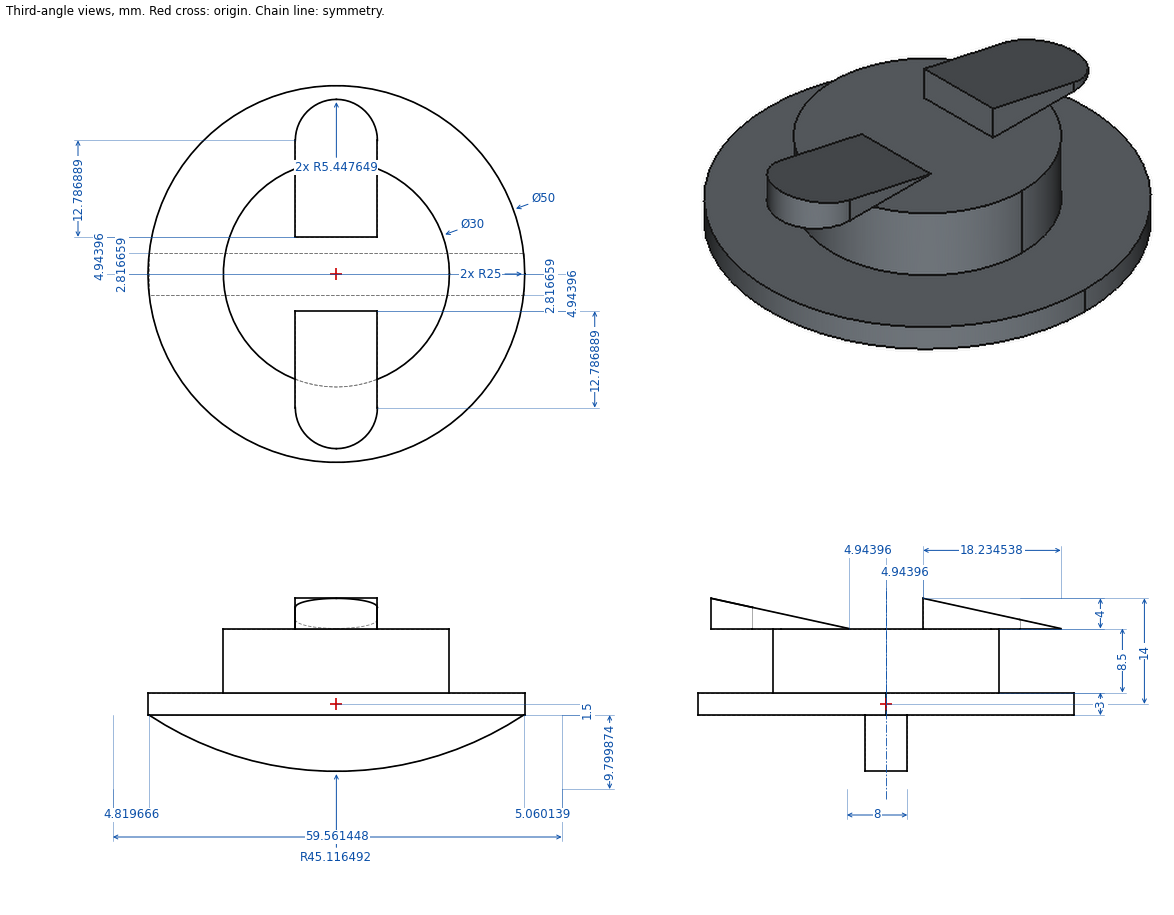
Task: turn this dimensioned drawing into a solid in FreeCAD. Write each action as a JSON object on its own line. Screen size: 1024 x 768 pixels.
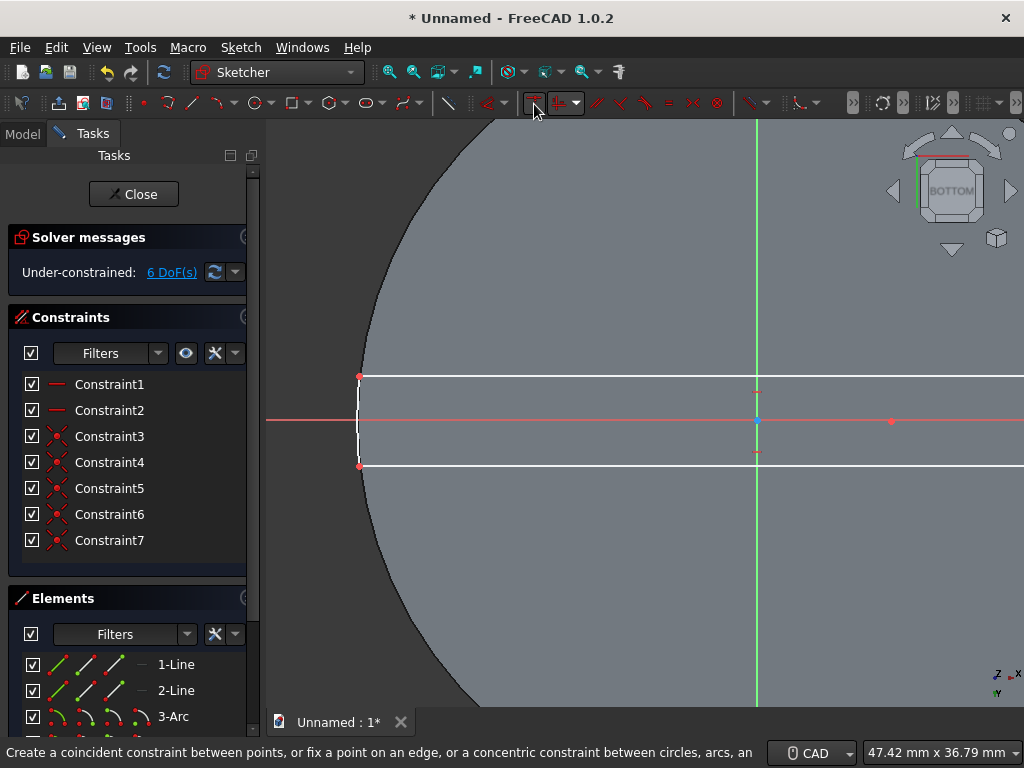
{"action": "left_click_drag", "start_coordinate": [747, 410], "coordinate": [901, 431]}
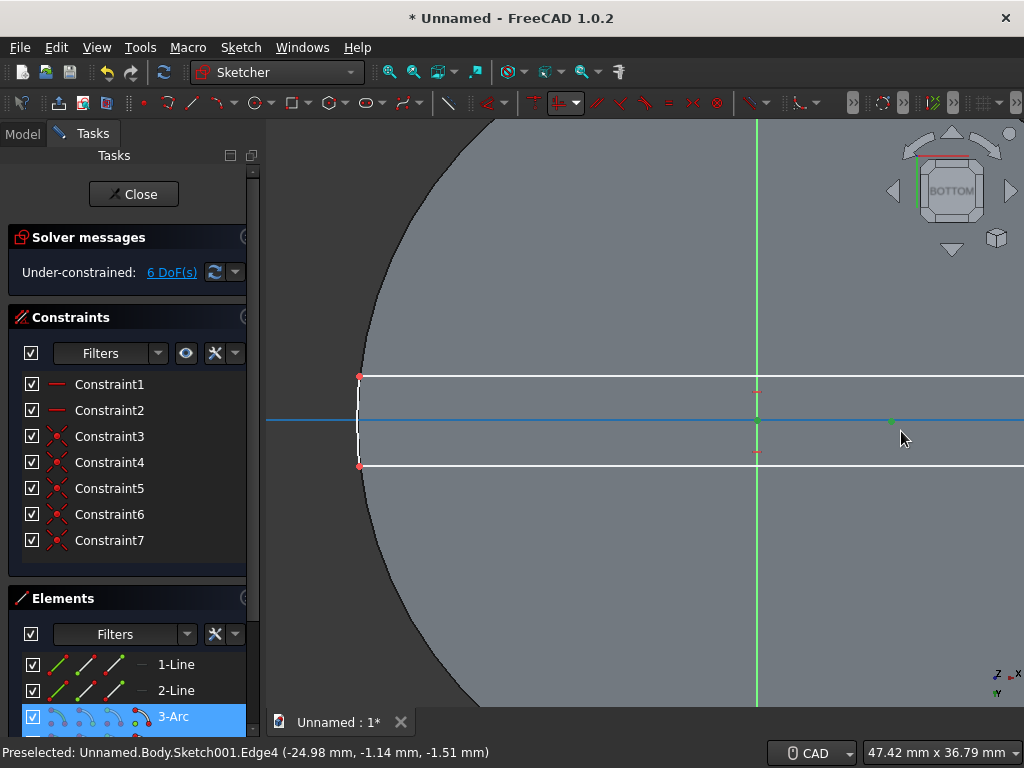
{"action": "left_click", "coordinate": [534, 104]}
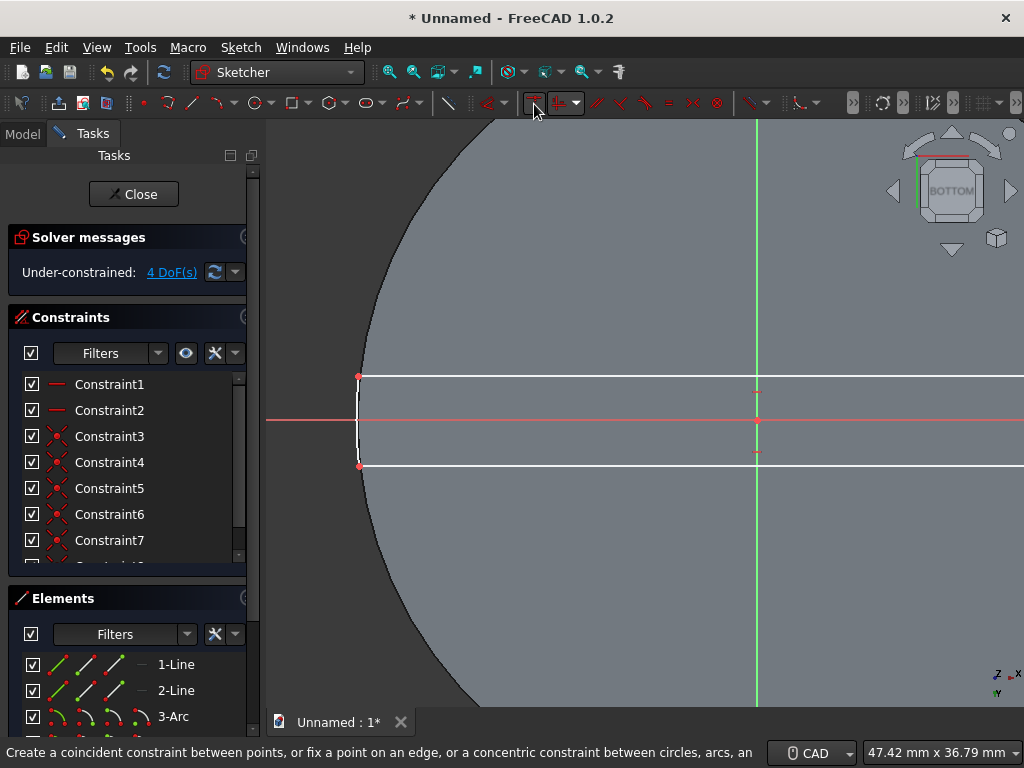
{"action": "left_click", "coordinate": [488, 104]}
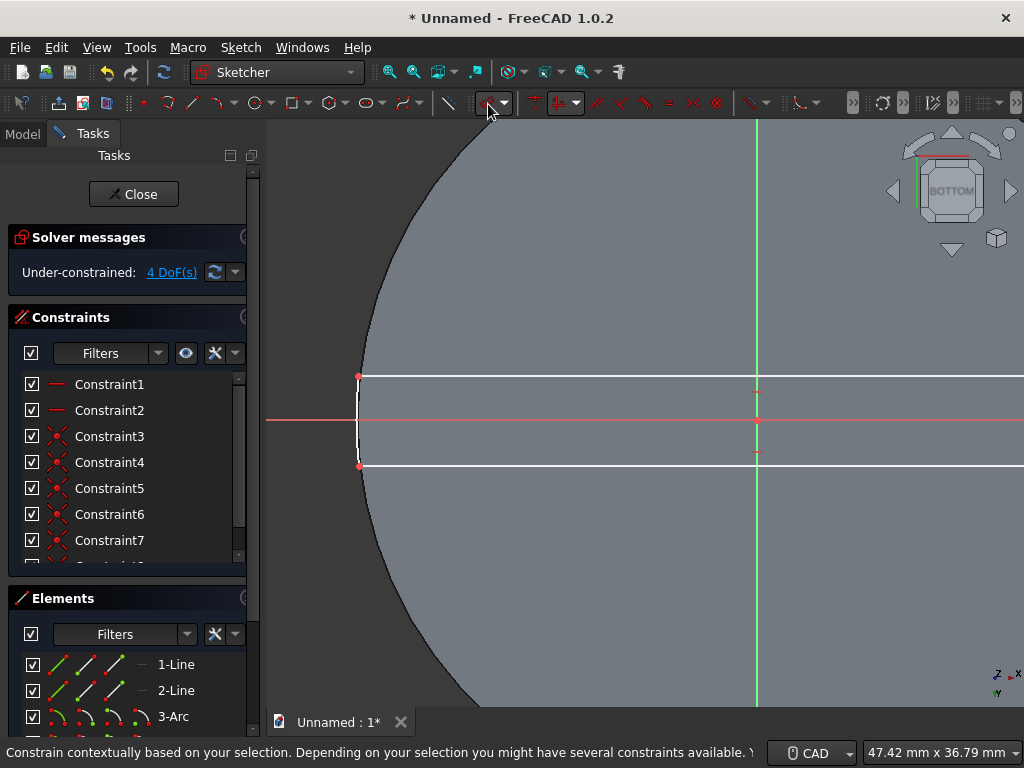
{"action": "scroll", "coordinate": [357, 404], "scroll_direction": "down", "scroll_amount": 3}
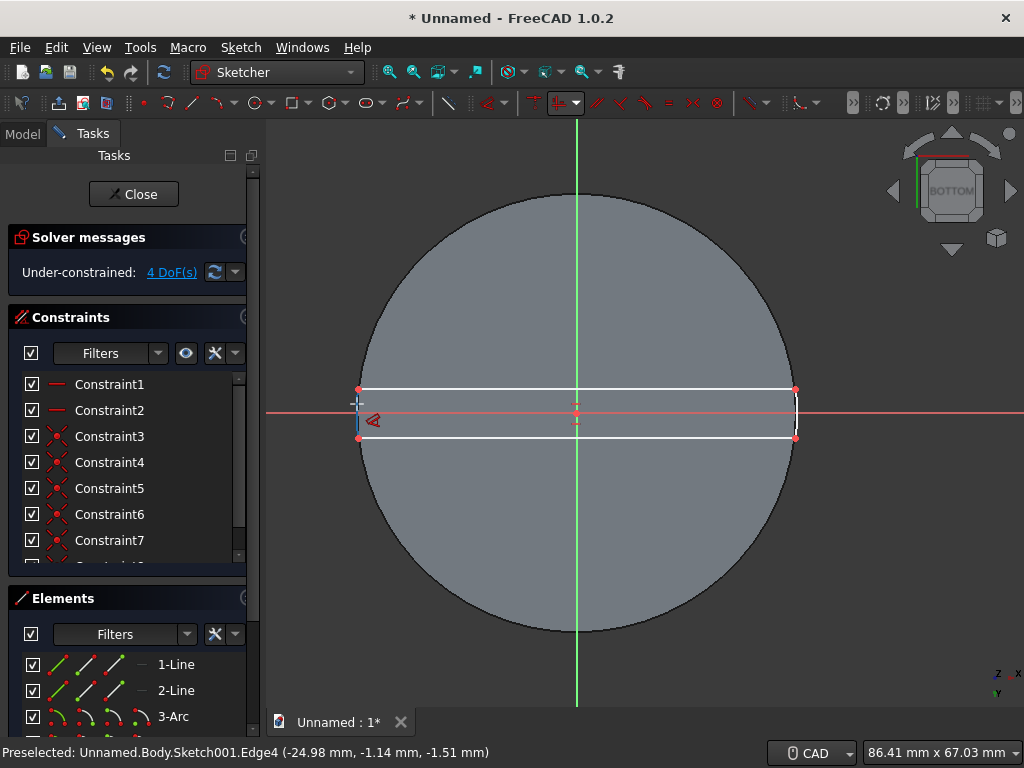
{"action": "scroll", "coordinate": [797, 424], "scroll_direction": "up", "scroll_amount": 2}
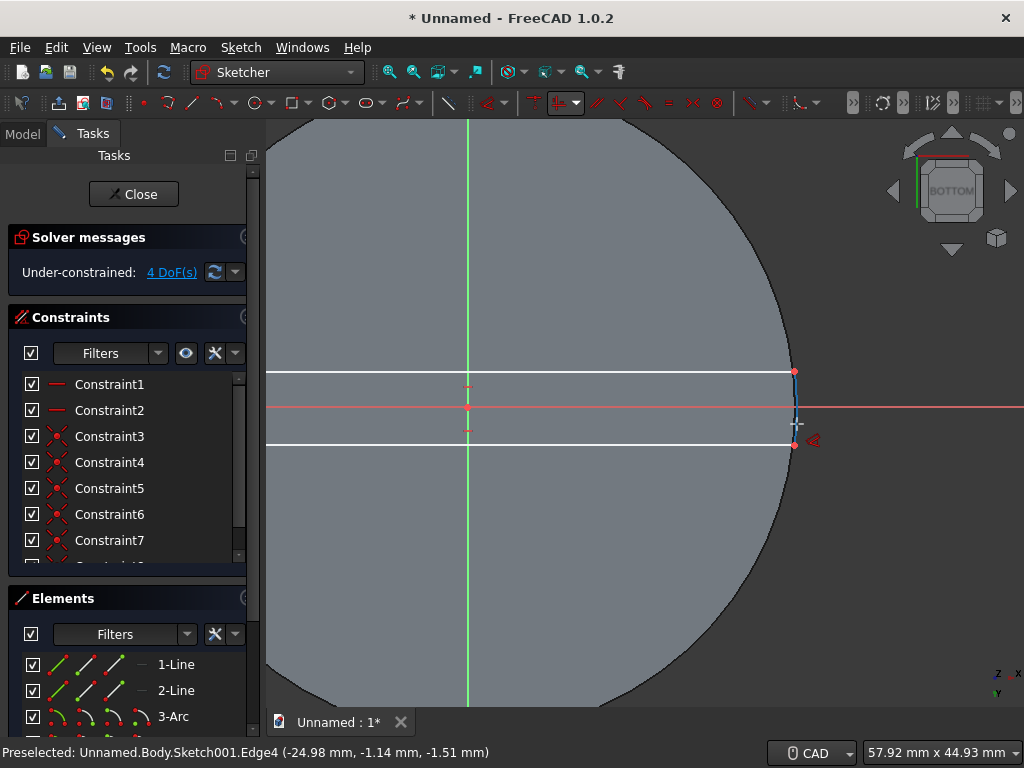
{"action": "left_click", "coordinate": [796, 423]}
{"action": "left_click", "coordinate": [828, 425]}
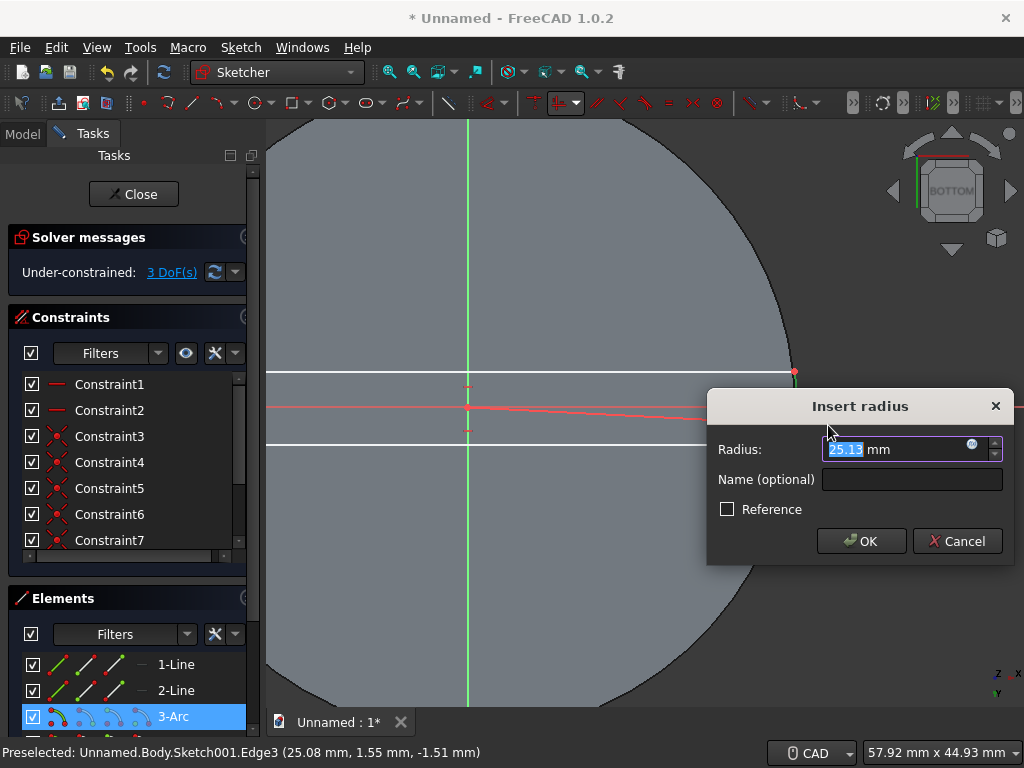
{"action": "type", "text": "25"}
{"action": "key", "text": "Return"}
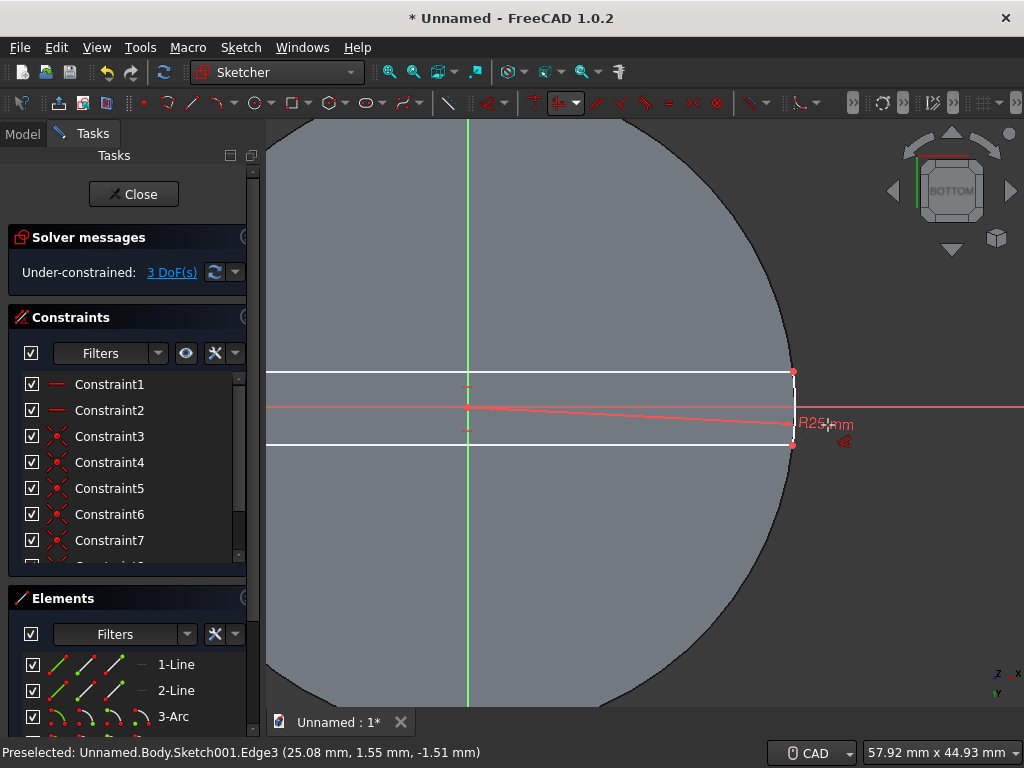
{"action": "scroll", "coordinate": [797, 424], "scroll_direction": "down", "scroll_amount": 2}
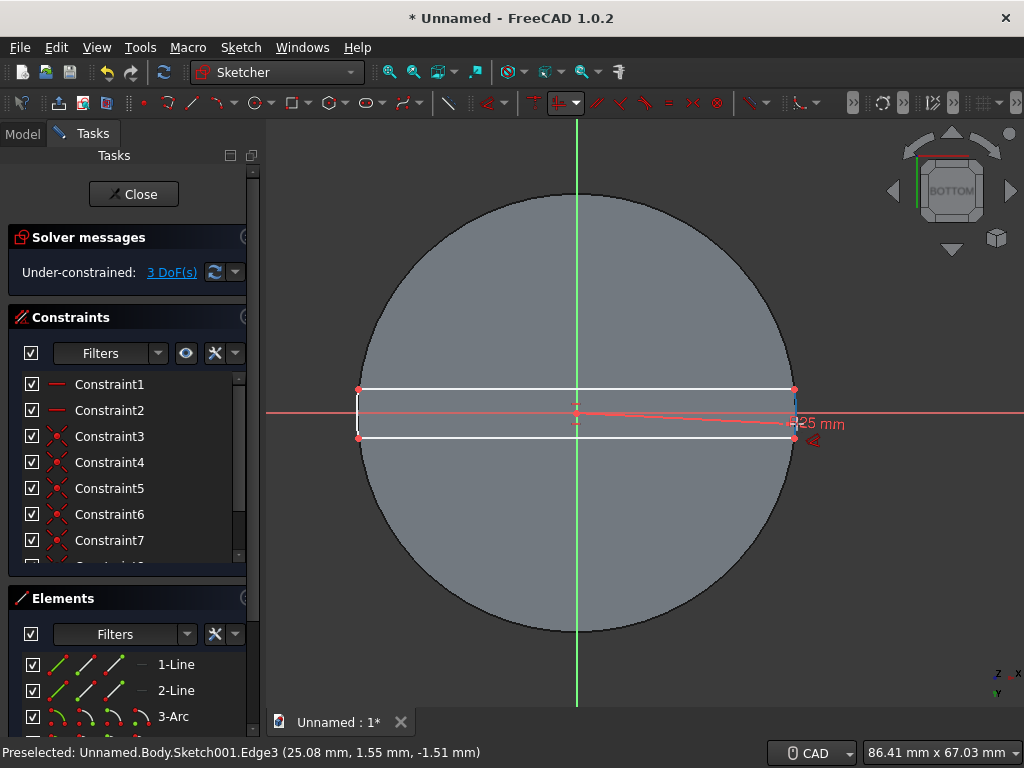
{"action": "scroll", "coordinate": [357, 404], "scroll_direction": "up", "scroll_amount": 3}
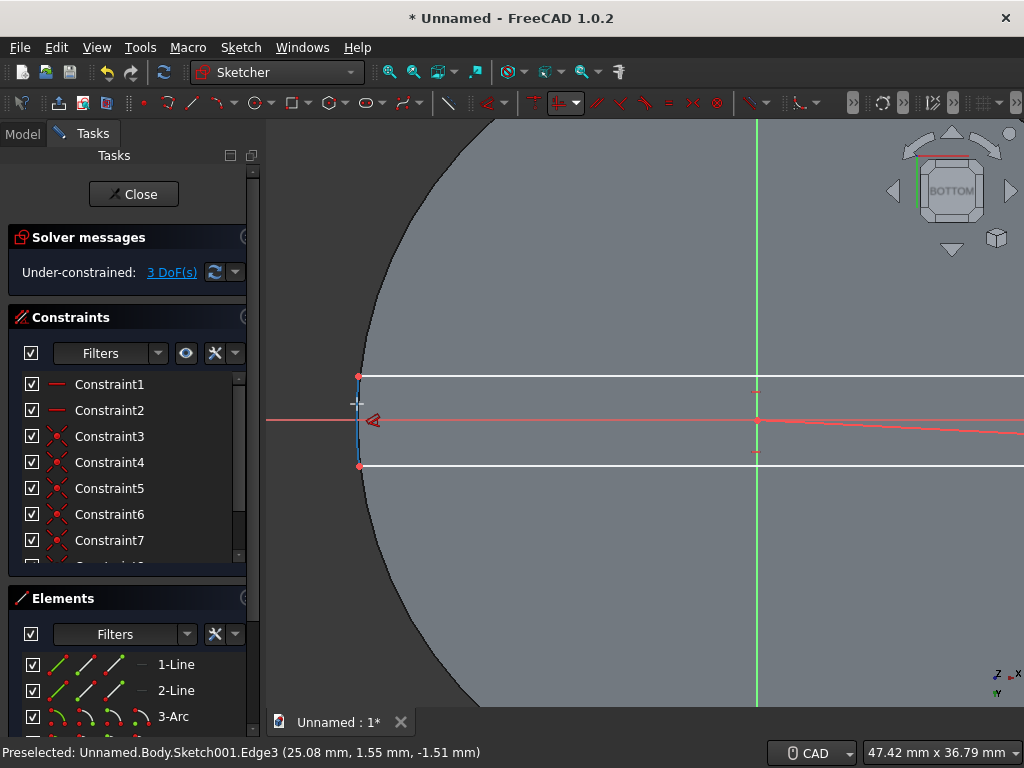
{"action": "left_click", "coordinate": [357, 403]}
{"action": "left_click", "coordinate": [325, 402]}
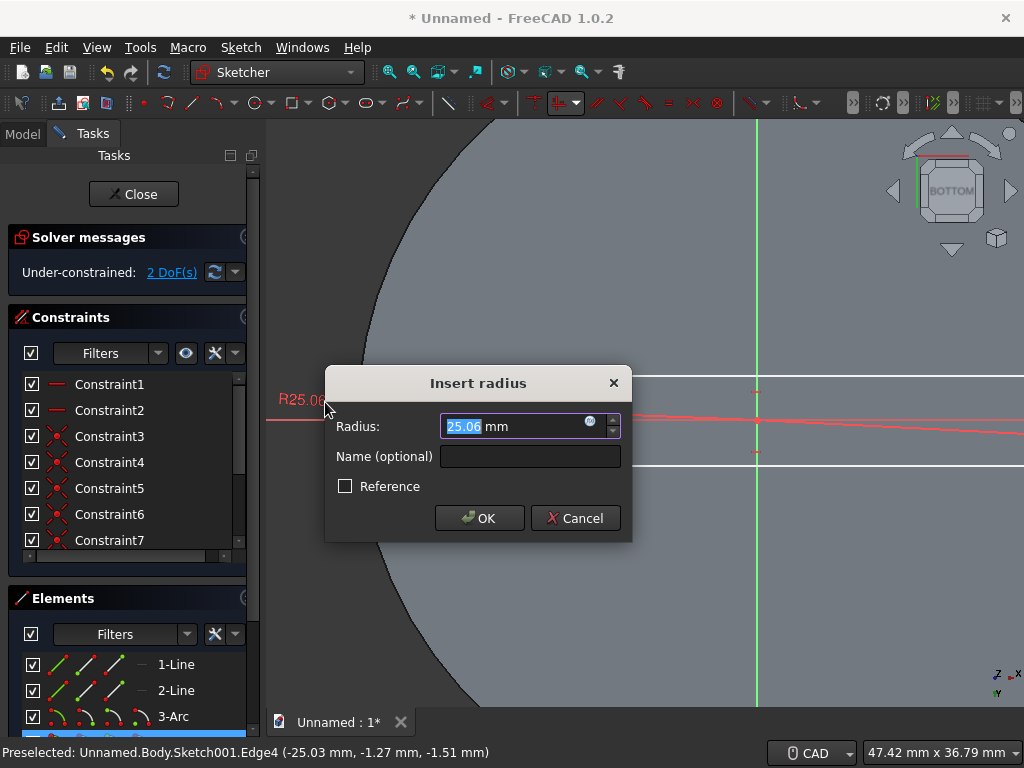
{"action": "type", "text": "25"}
{"action": "key", "text": "Return"}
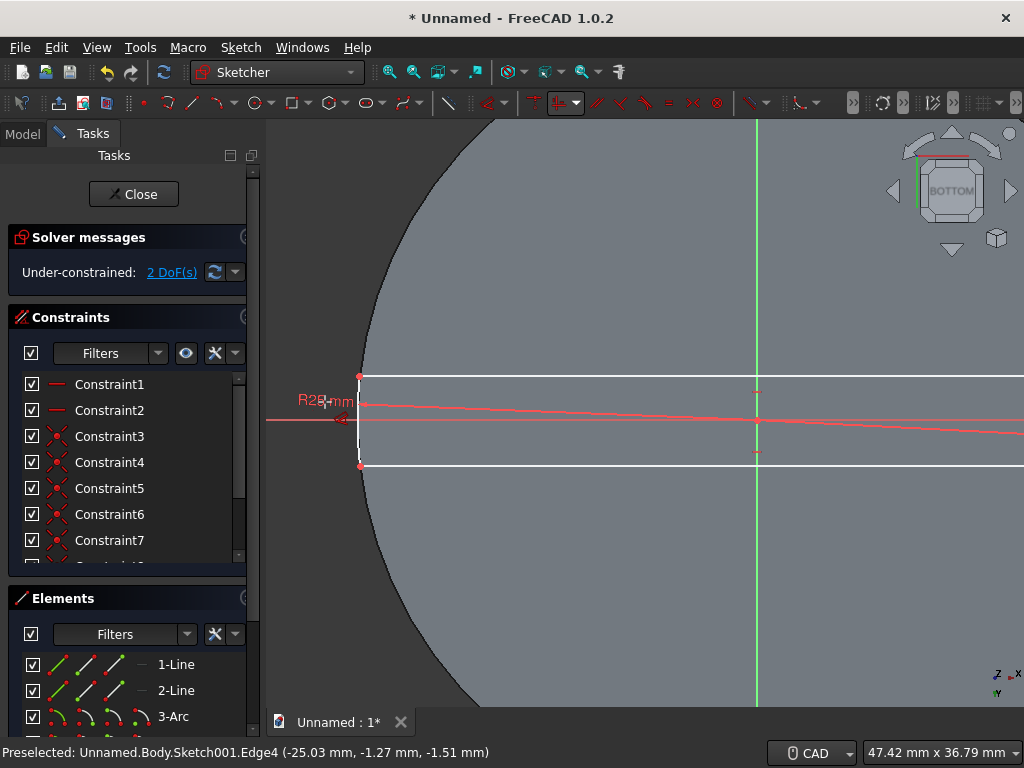
{"action": "left_click", "coordinate": [360, 466]}
{"action": "left_click", "coordinate": [326, 443]}